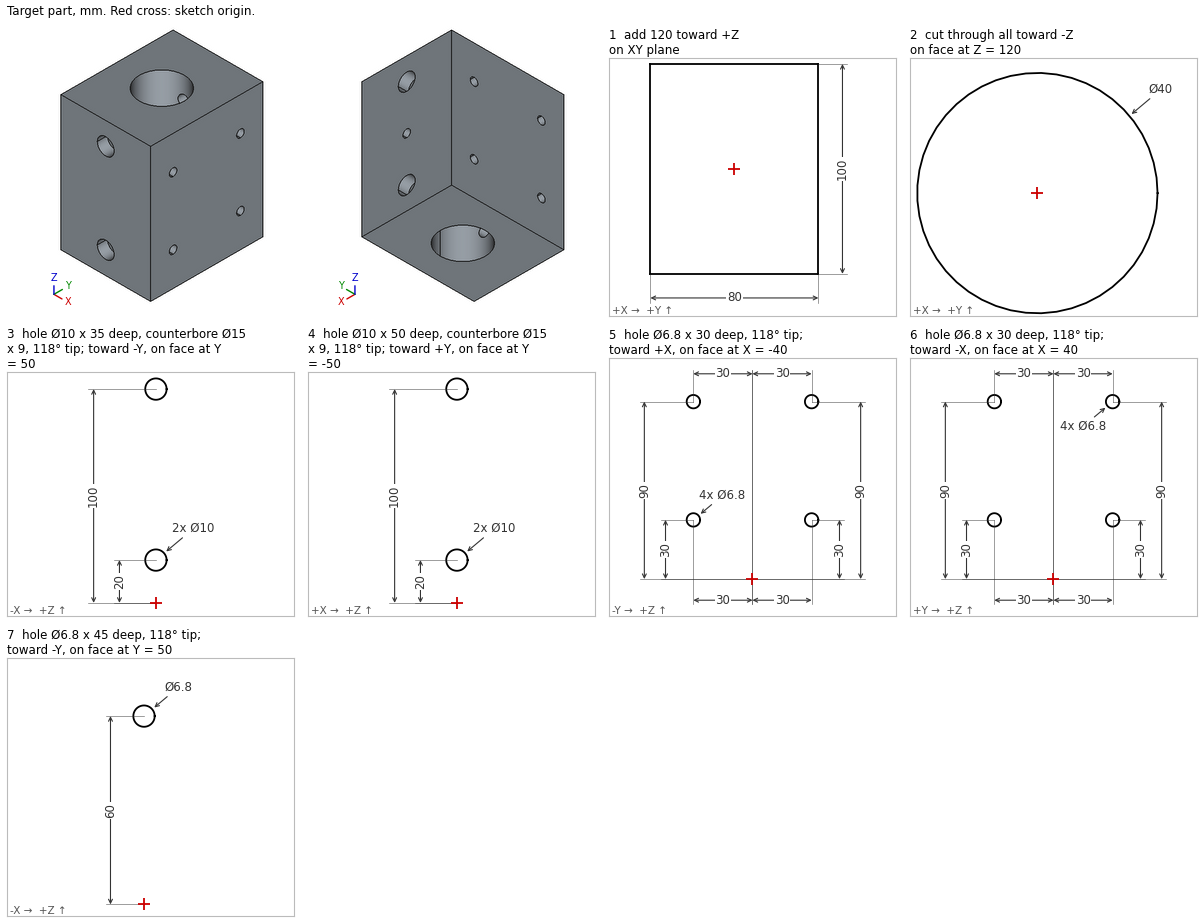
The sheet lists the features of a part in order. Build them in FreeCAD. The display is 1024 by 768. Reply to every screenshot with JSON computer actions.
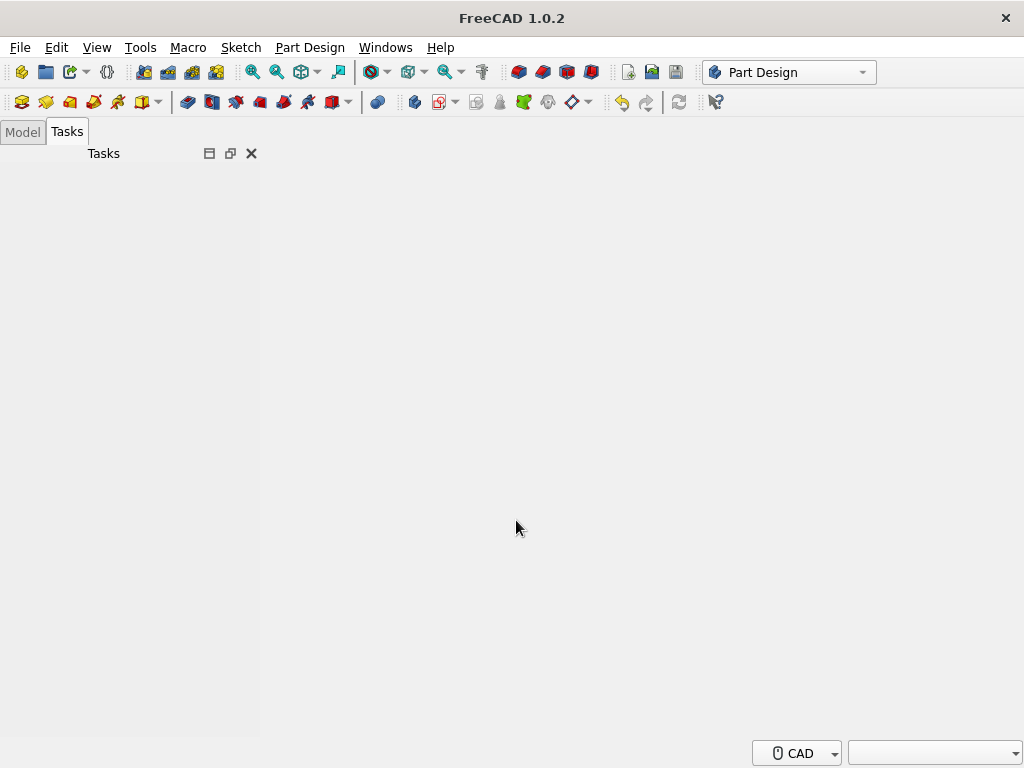
{"action": "left_click", "coordinate": [628, 72]}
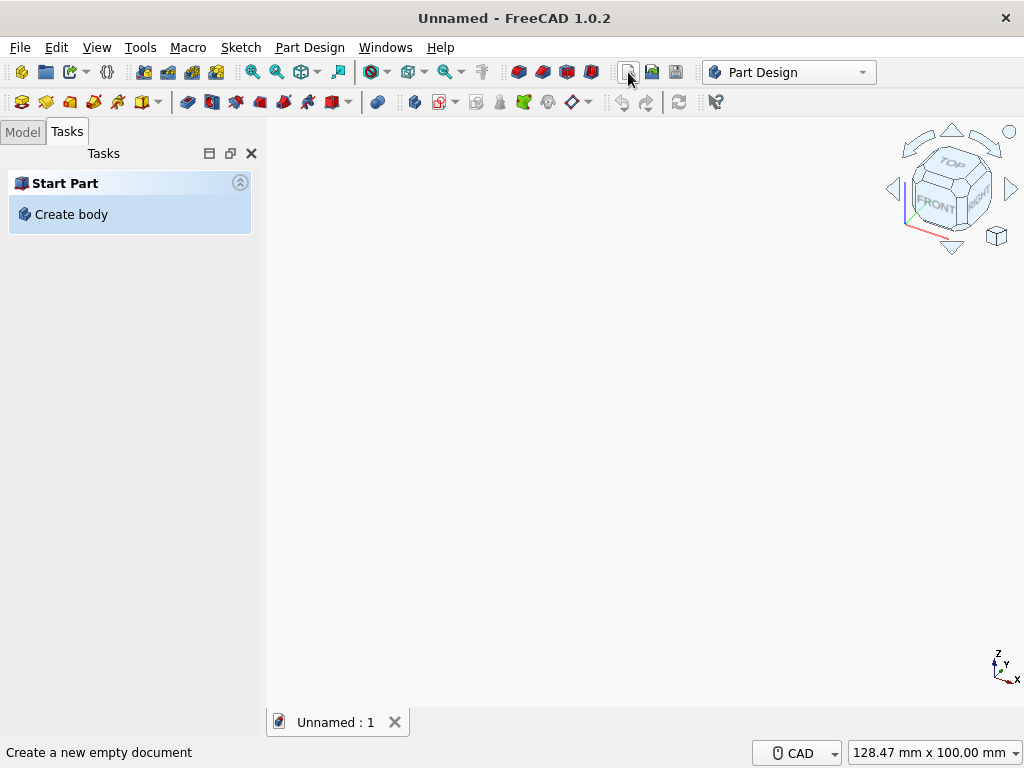
{"action": "left_click", "coordinate": [440, 102]}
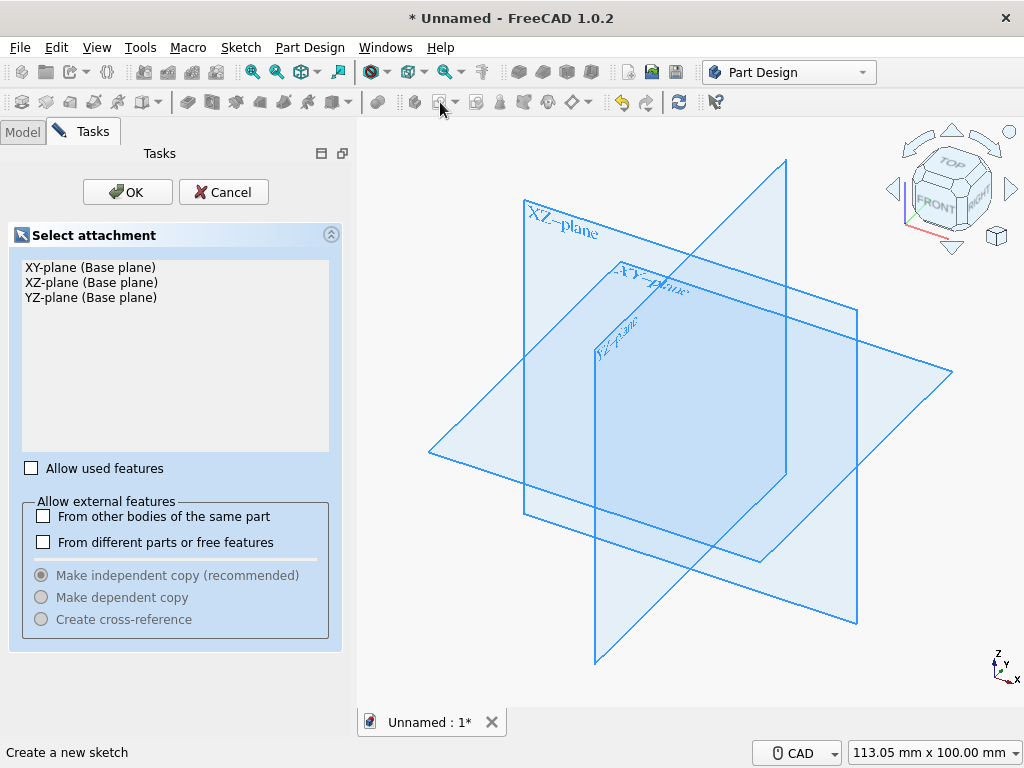
{"action": "left_click", "coordinate": [82, 268]}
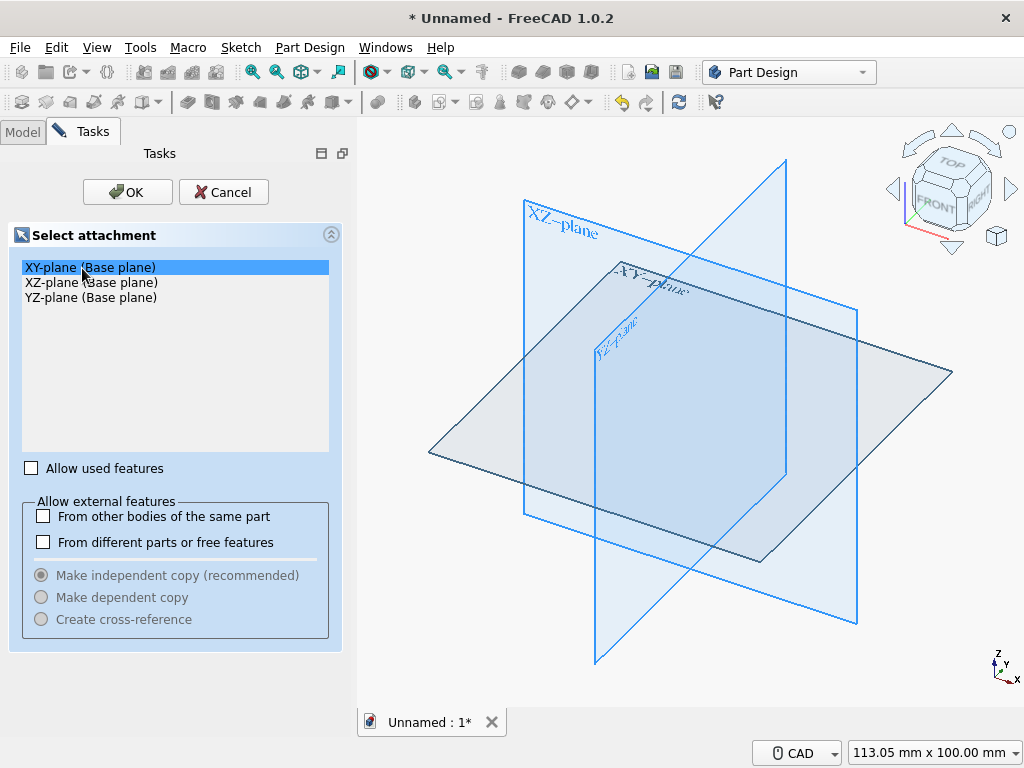
{"action": "left_click", "coordinate": [128, 192]}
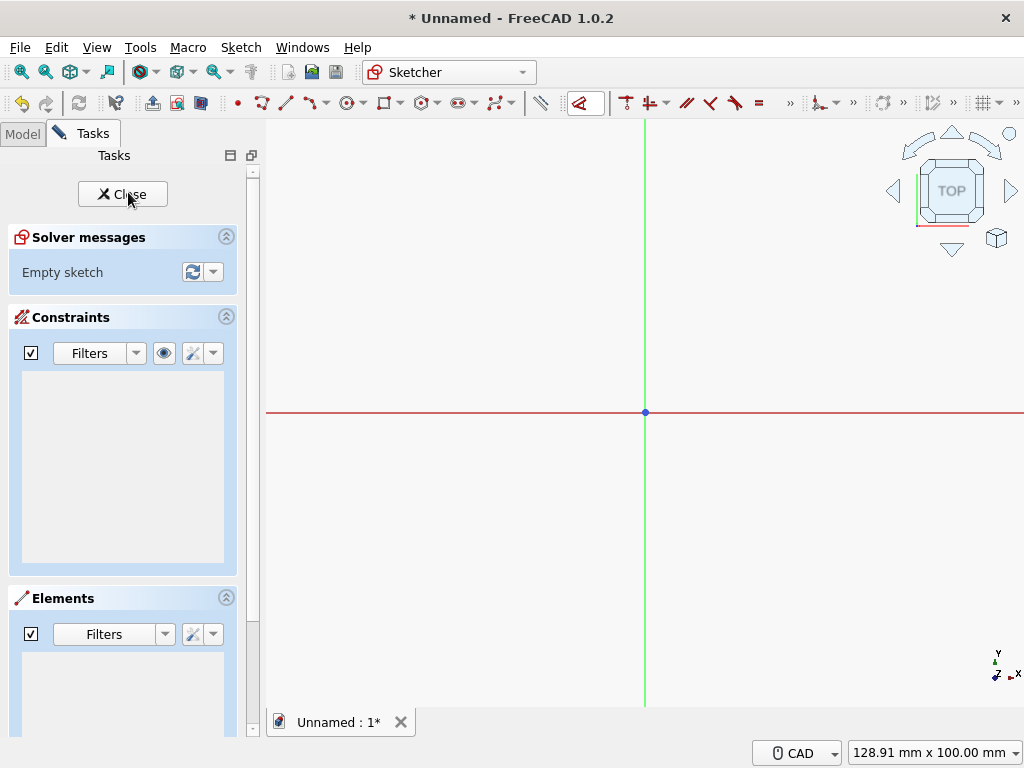
{"action": "scroll", "coordinate": [437, 413], "scroll_direction": "down", "scroll_amount": 2}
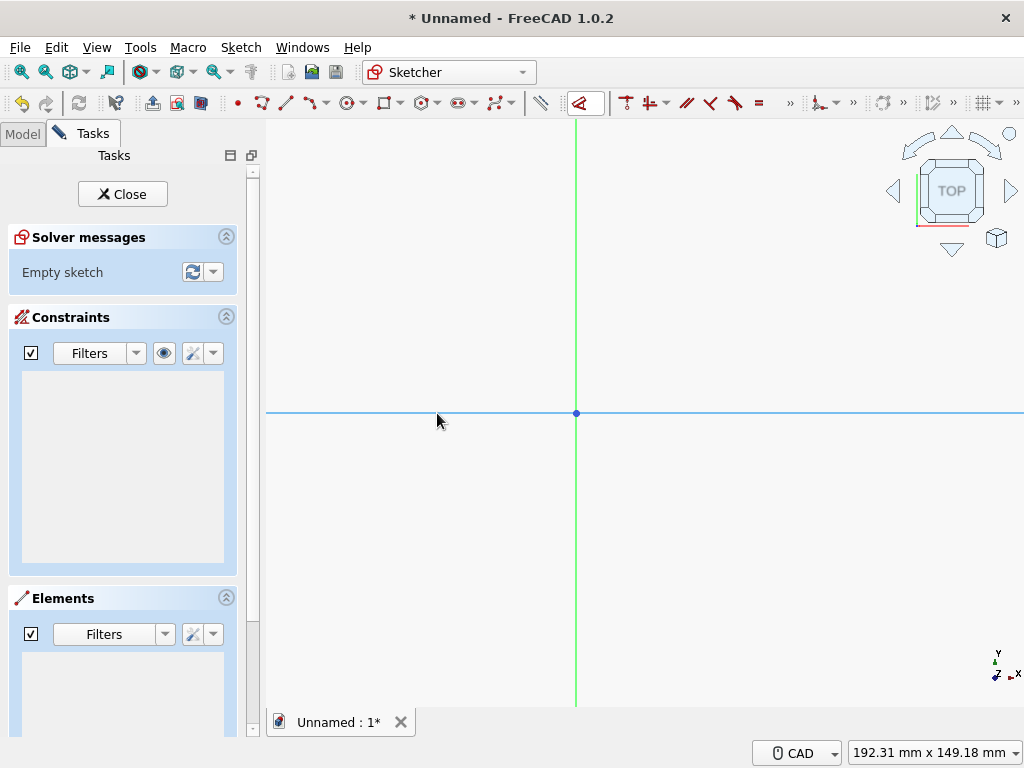
{"action": "key", "text": "g v"}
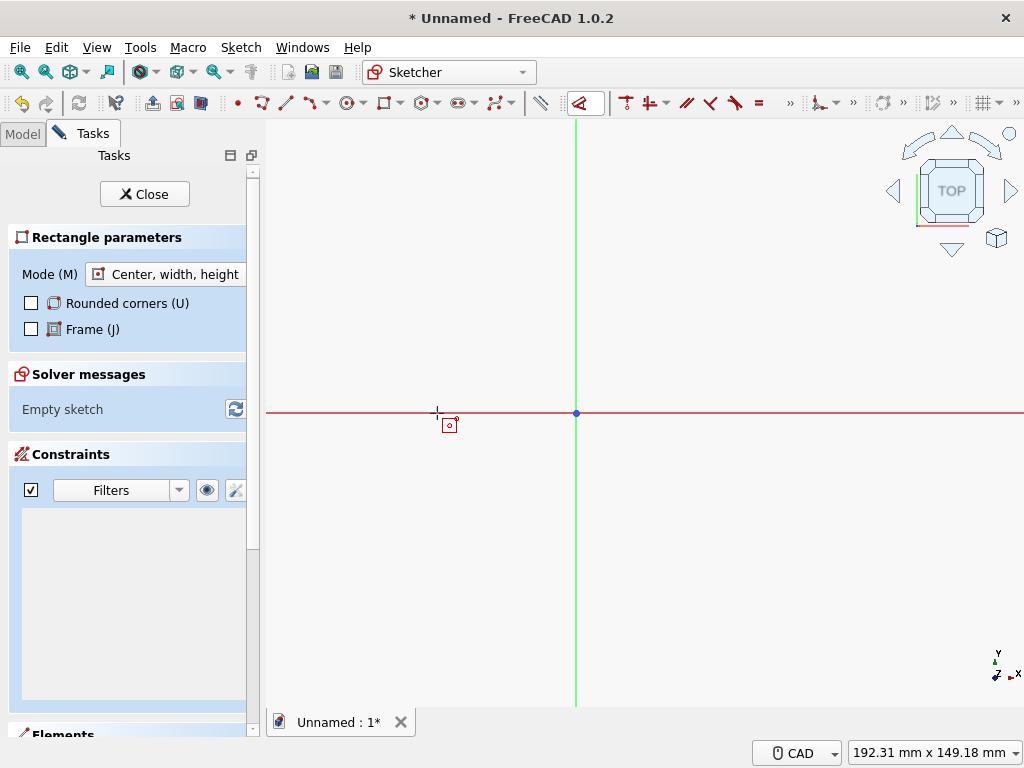
{"action": "left_click", "coordinate": [577, 413]}
{"action": "mouse_move", "coordinate": [734, 216]}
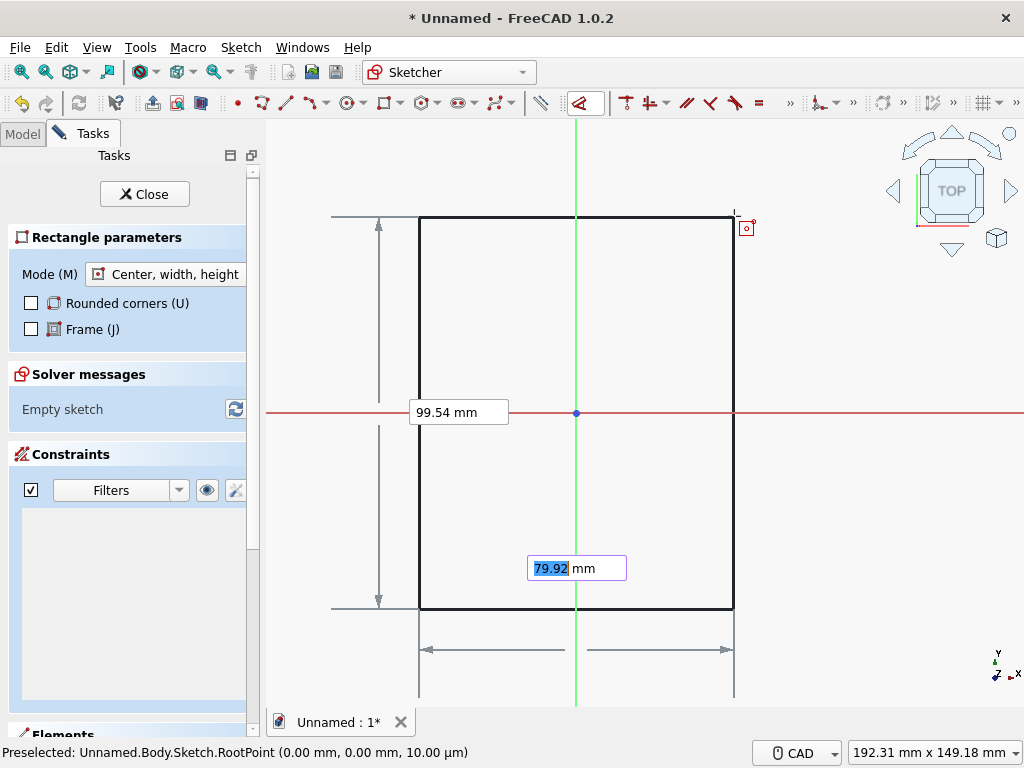
{"action": "type", "text": "80"}
{"action": "key", "text": "Tab"}
{"action": "type", "text": "100"}
{"action": "key", "text": "Return"}
{"action": "key", "text": "Escape"}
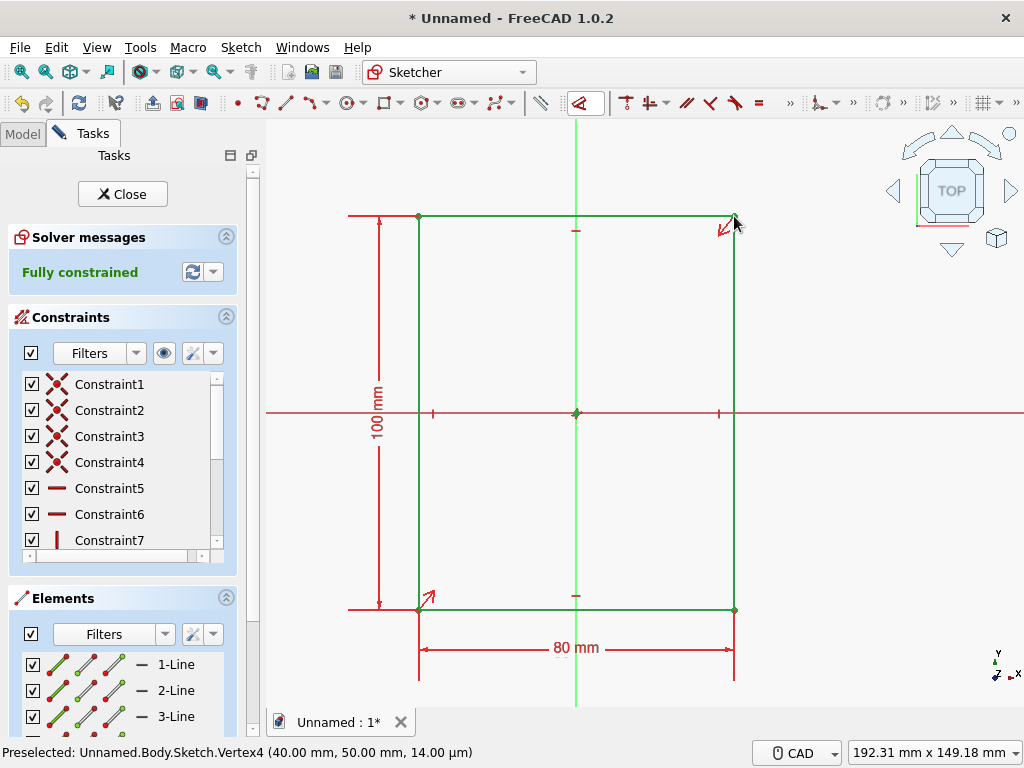
{"action": "left_click", "coordinate": [123, 194]}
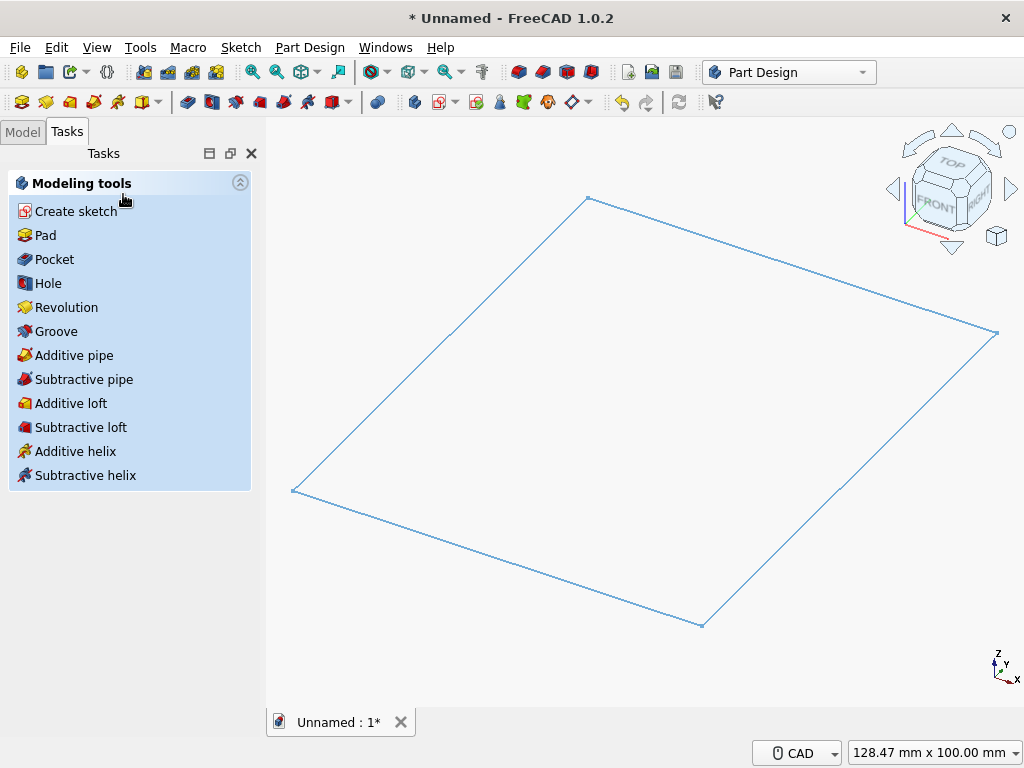
{"action": "left_click", "coordinate": [22, 102]}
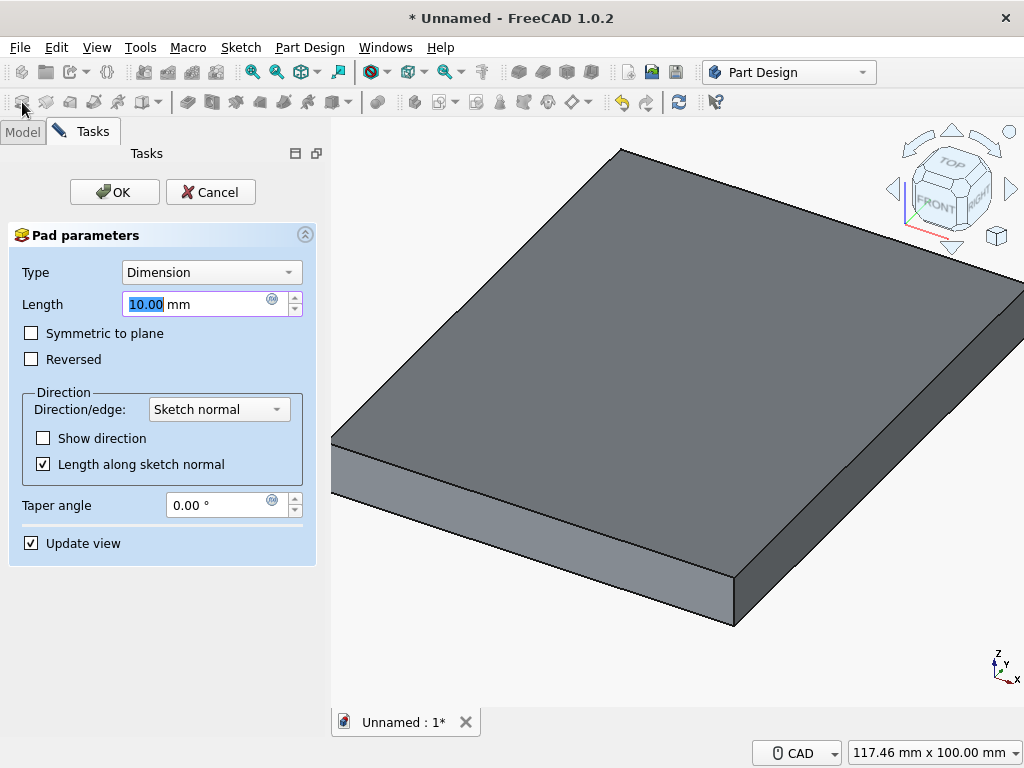
{"action": "type", "text": "120"}
{"action": "key", "text": "Tab"}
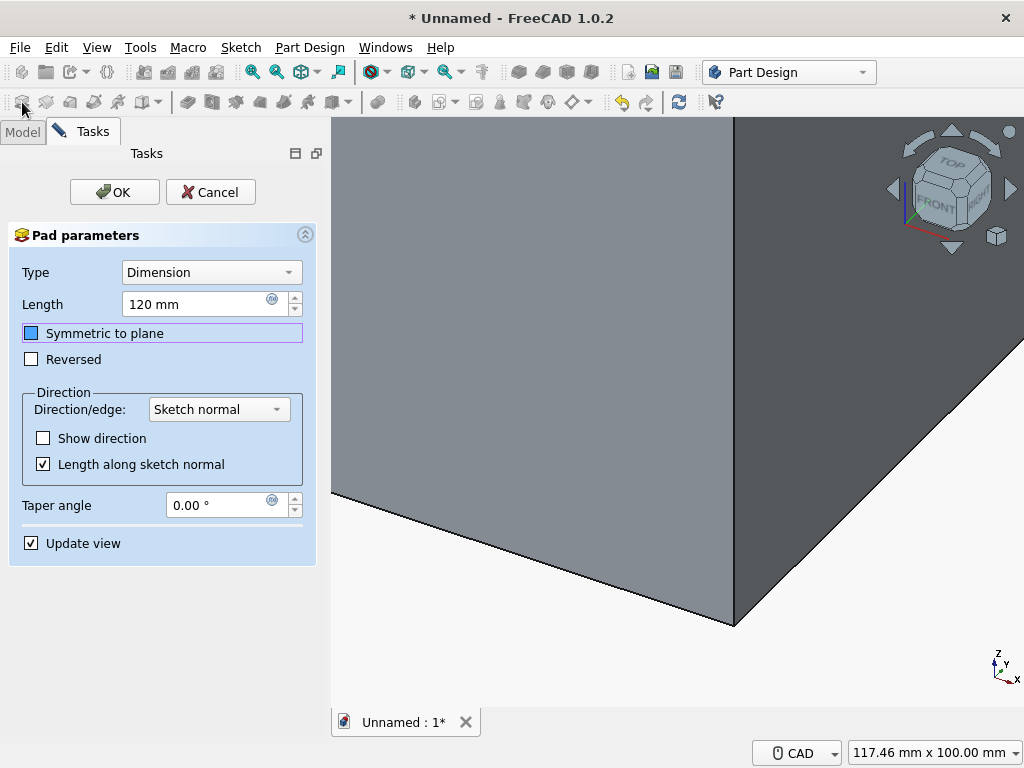
{"action": "left_click", "coordinate": [115, 192]}